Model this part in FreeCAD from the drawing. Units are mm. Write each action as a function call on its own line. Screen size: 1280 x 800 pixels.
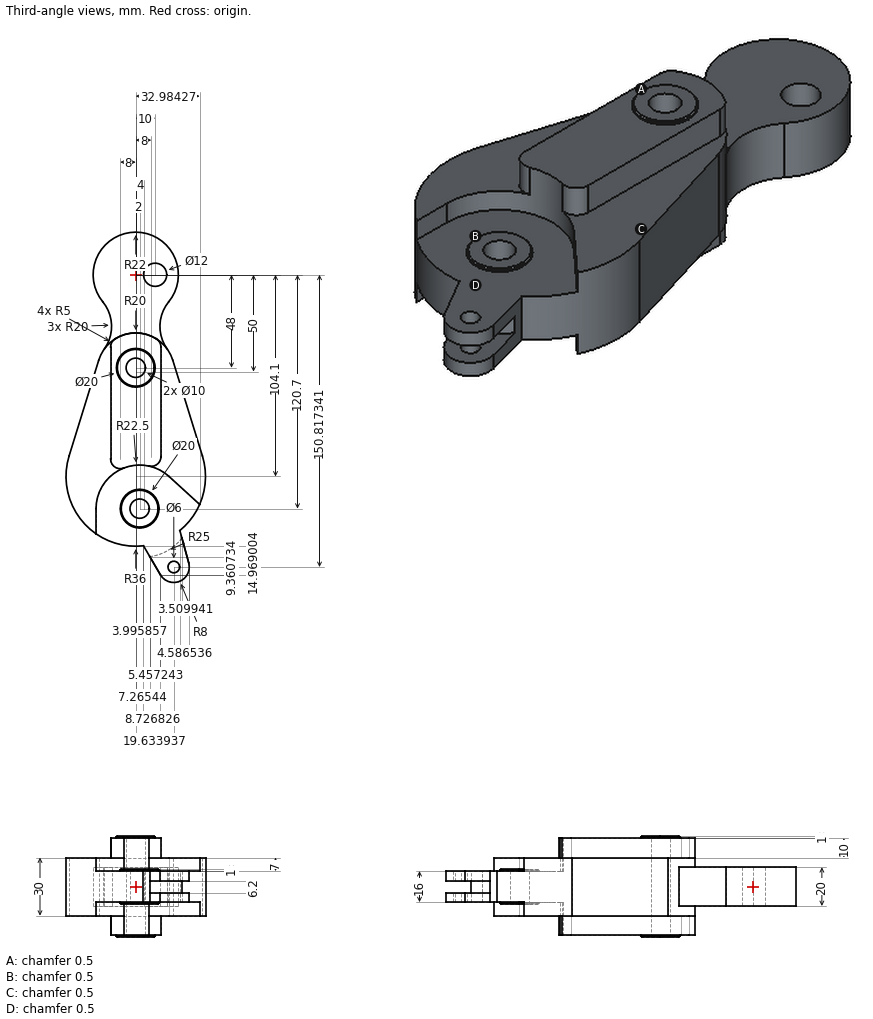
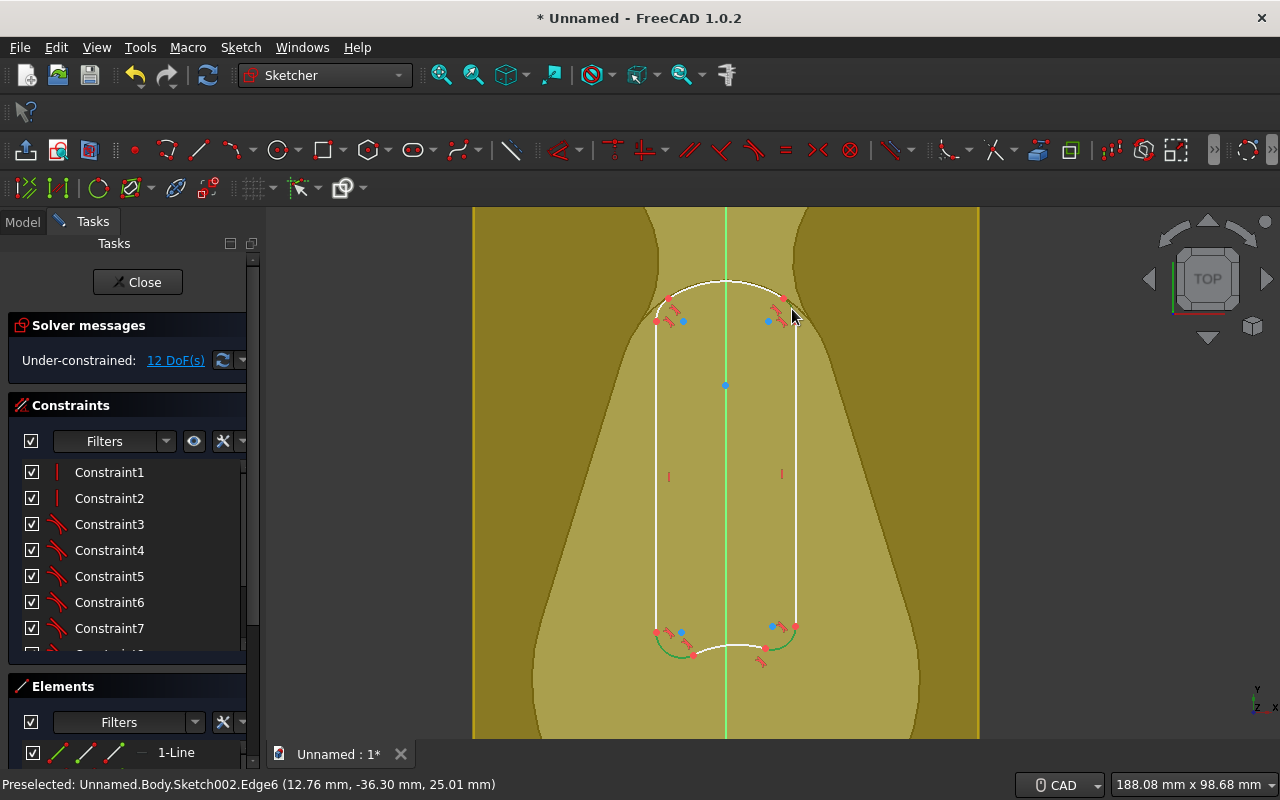
click(659, 309)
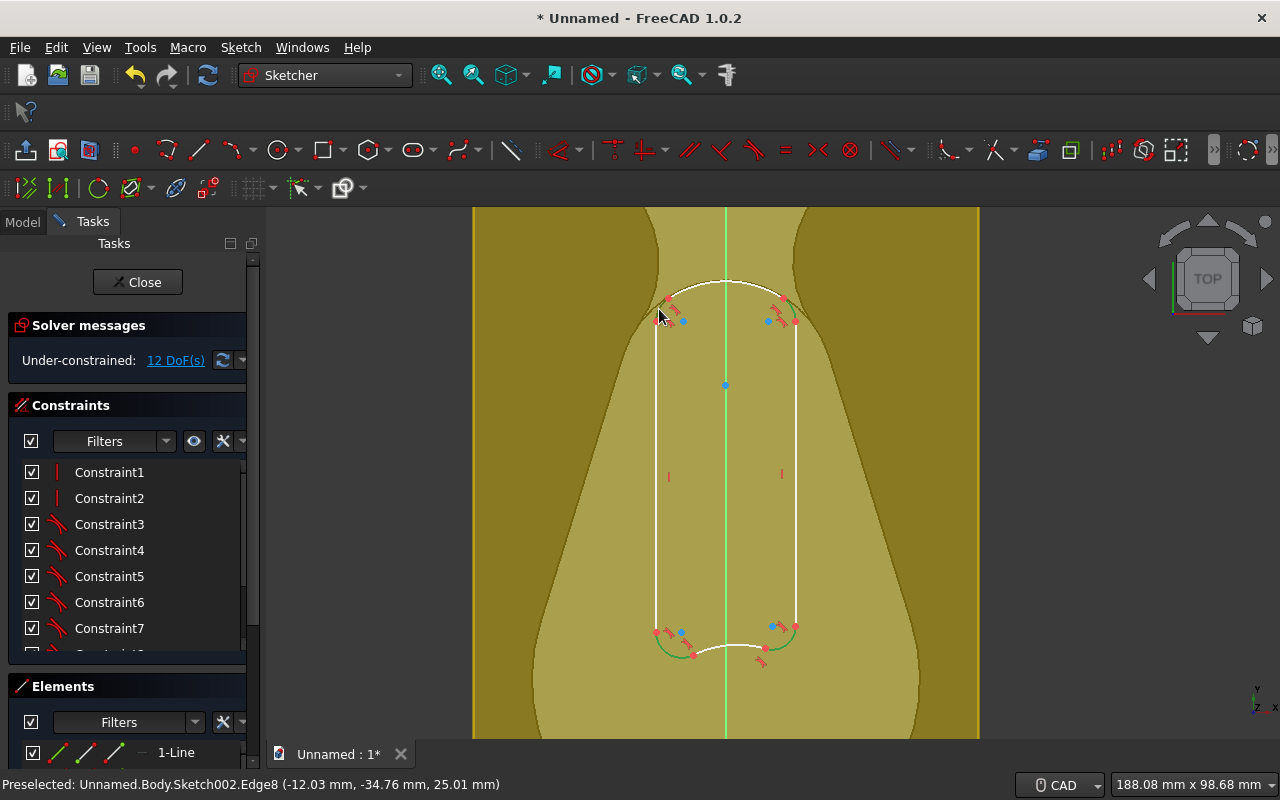
click(786, 150)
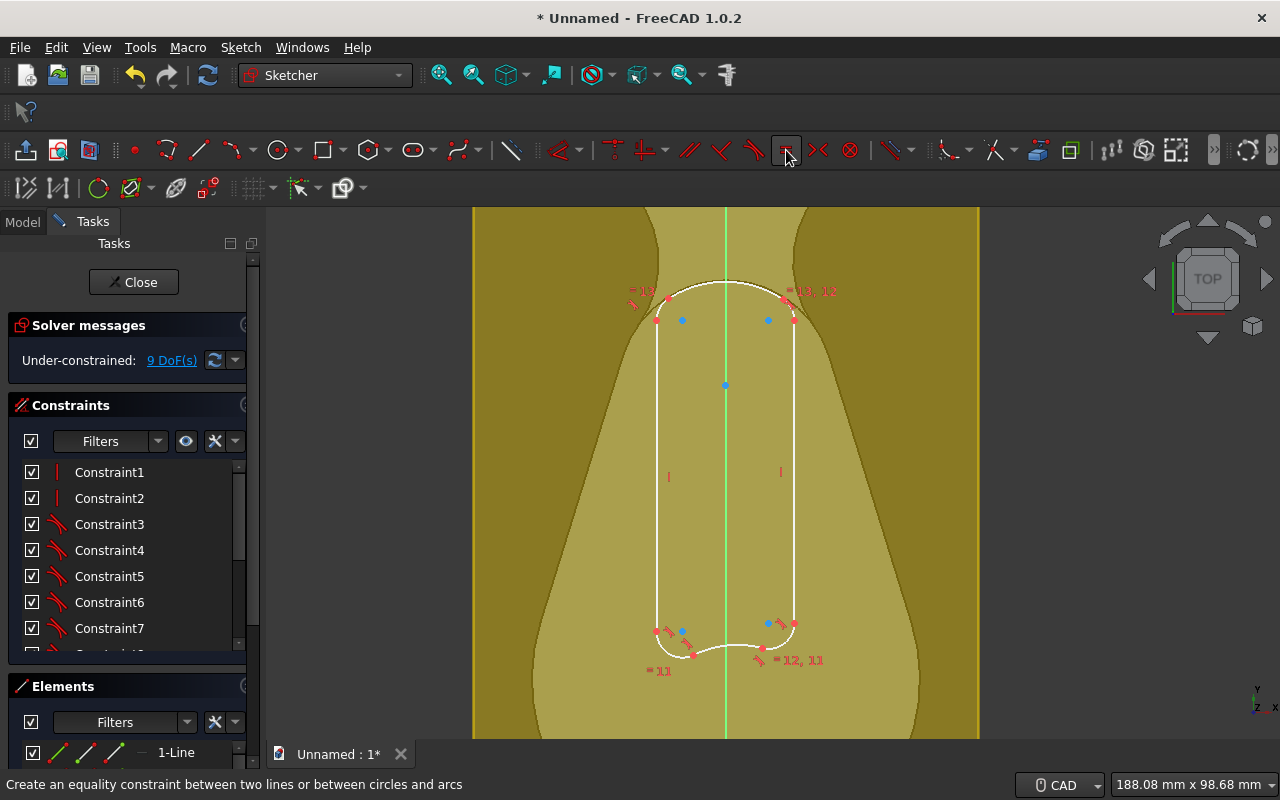
click(725, 385)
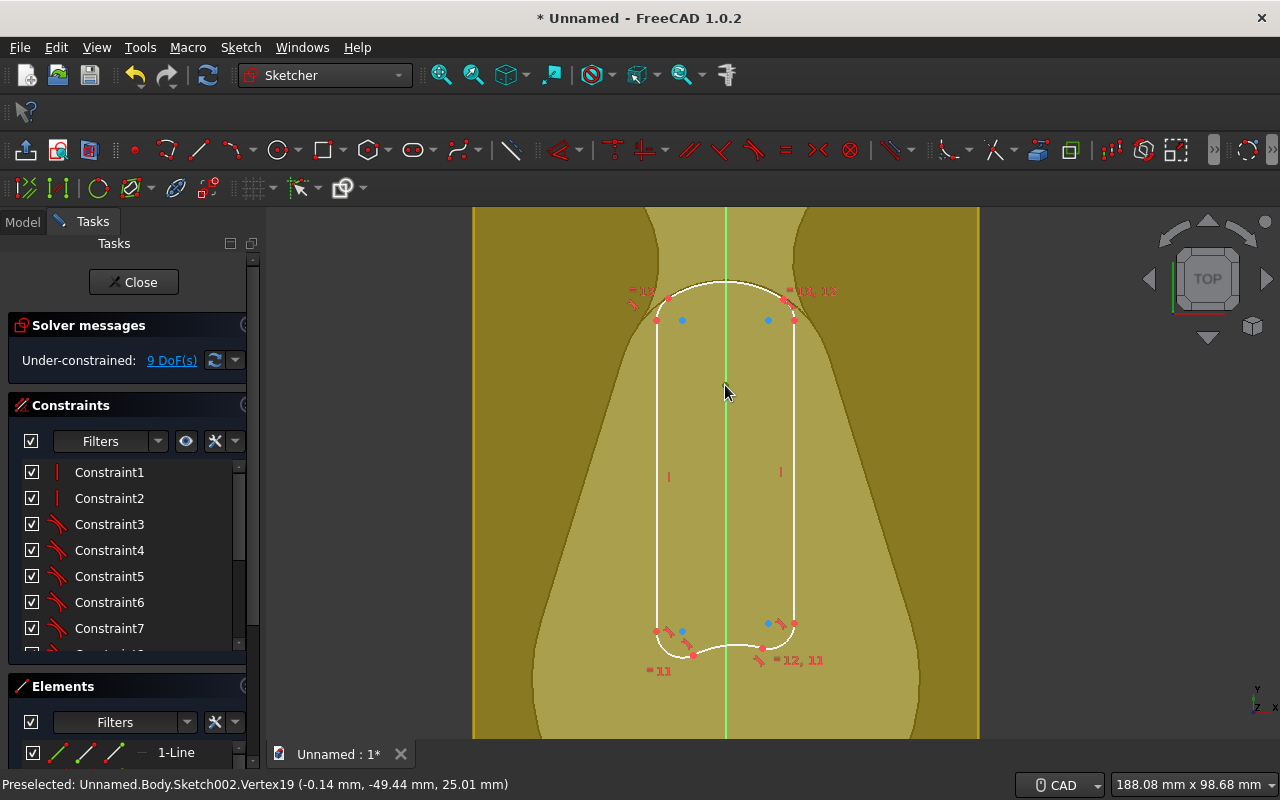
click(726, 677)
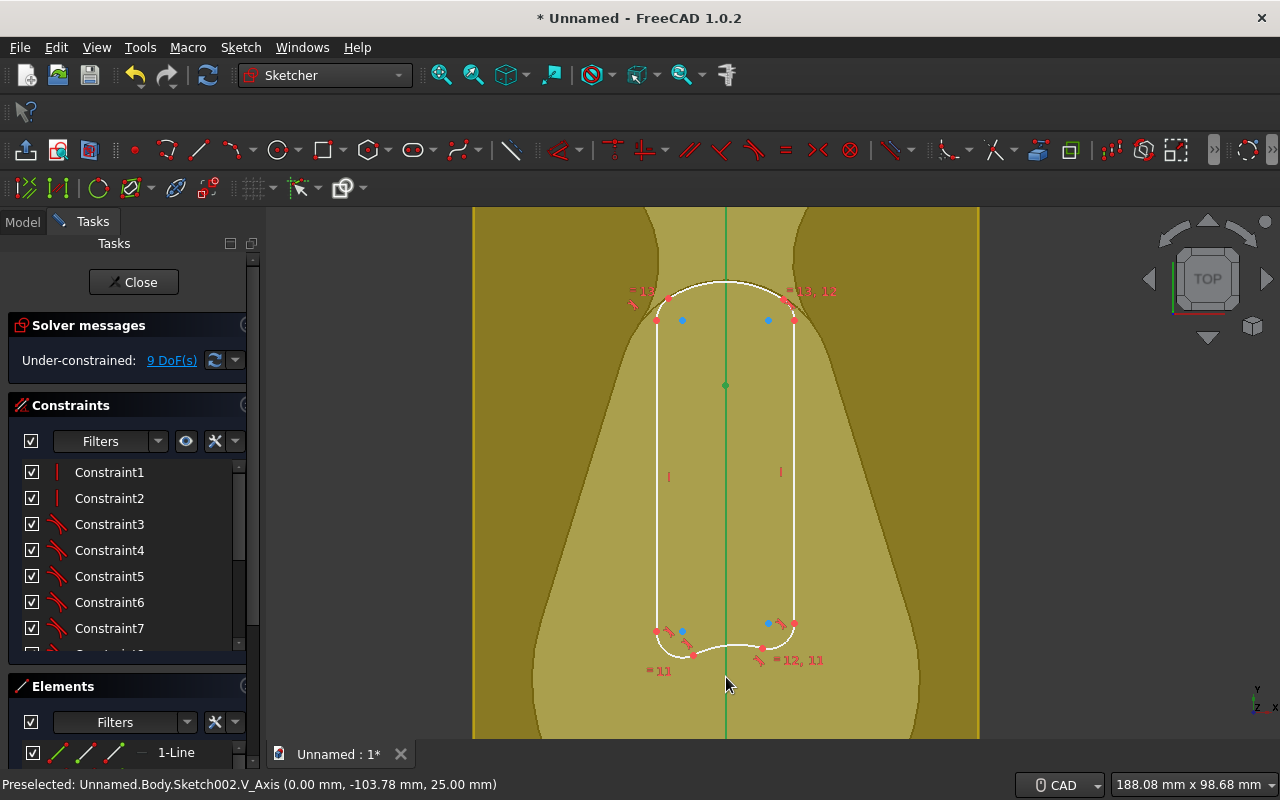
click(614, 150)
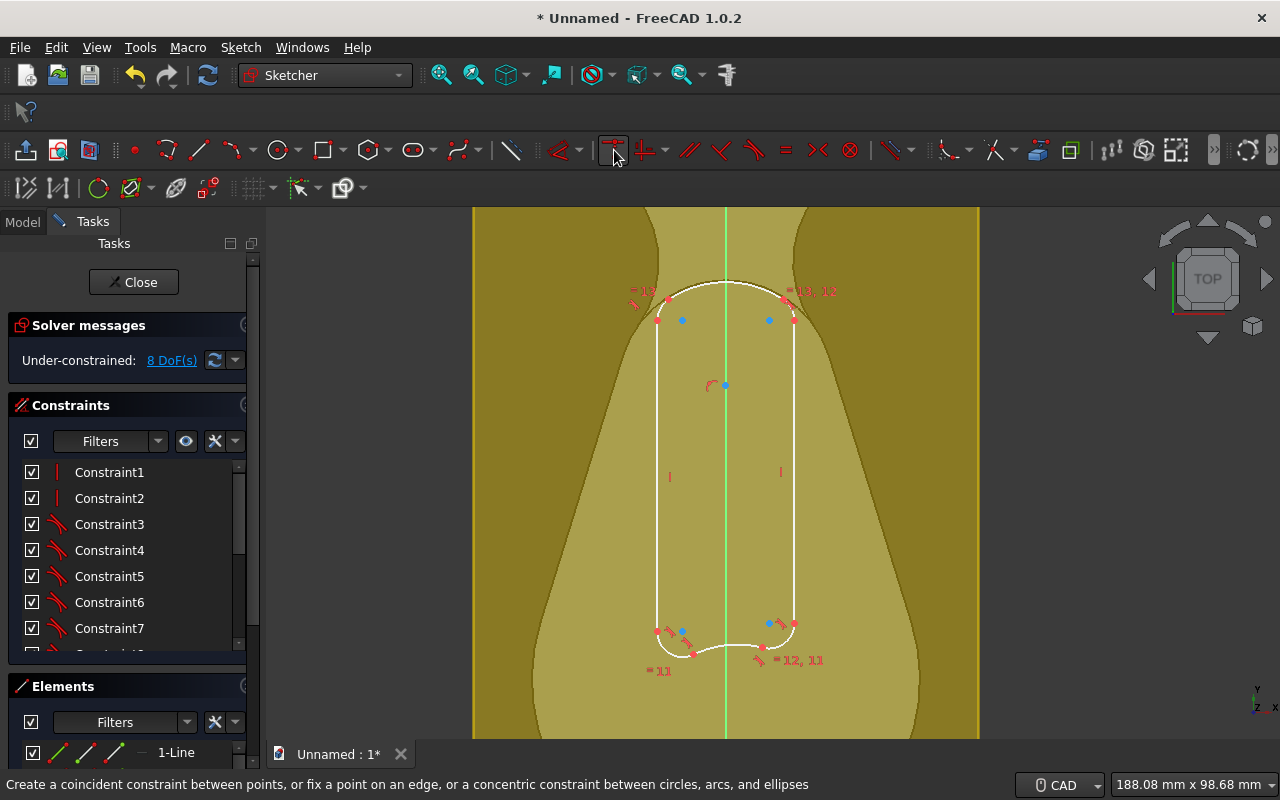
click(558, 150)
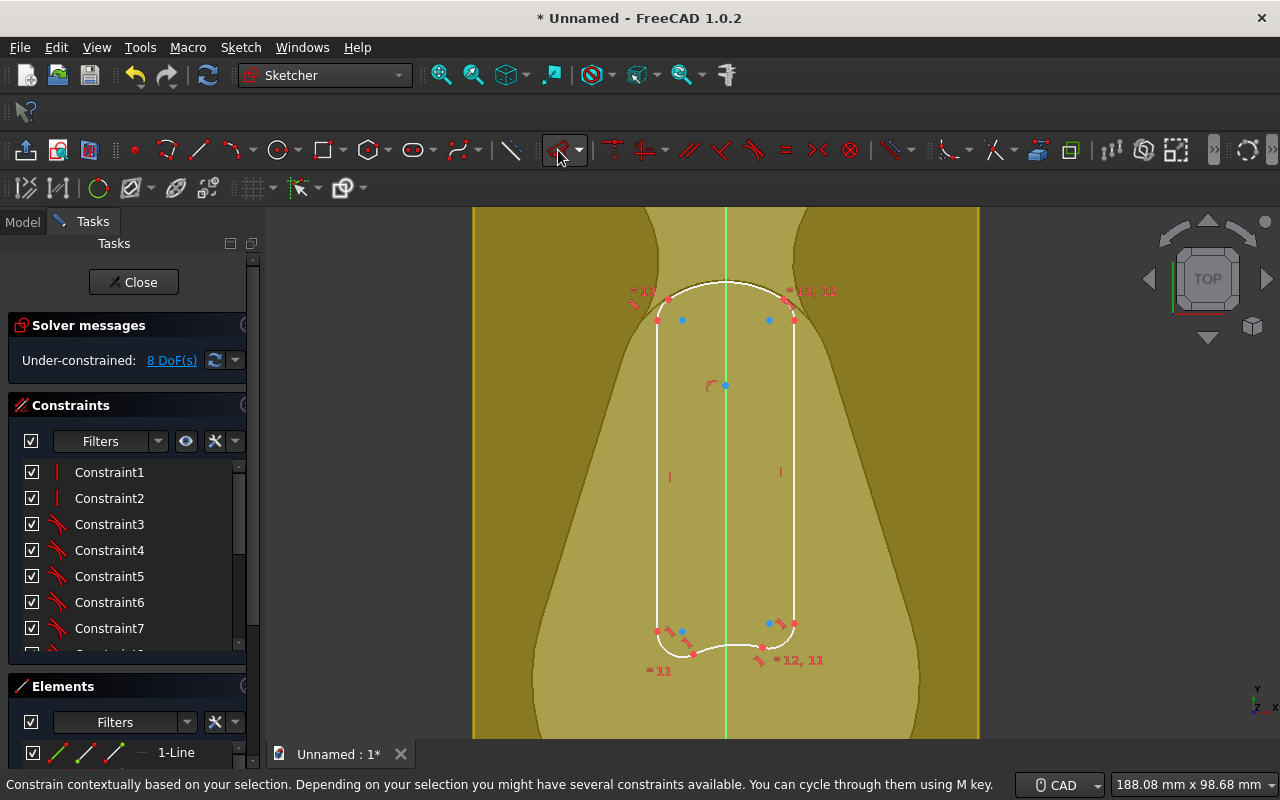
scroll(662, 646, up, 2)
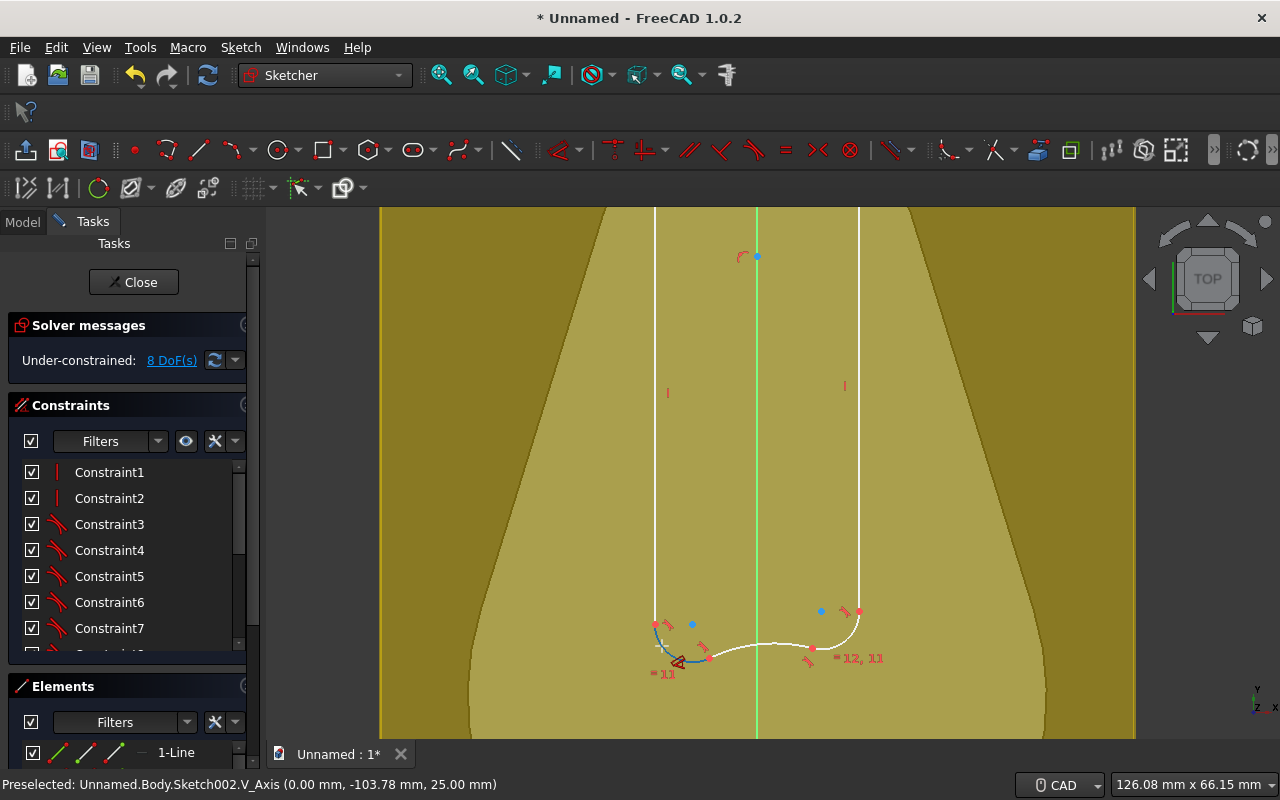
click(662, 646)
click(636, 664)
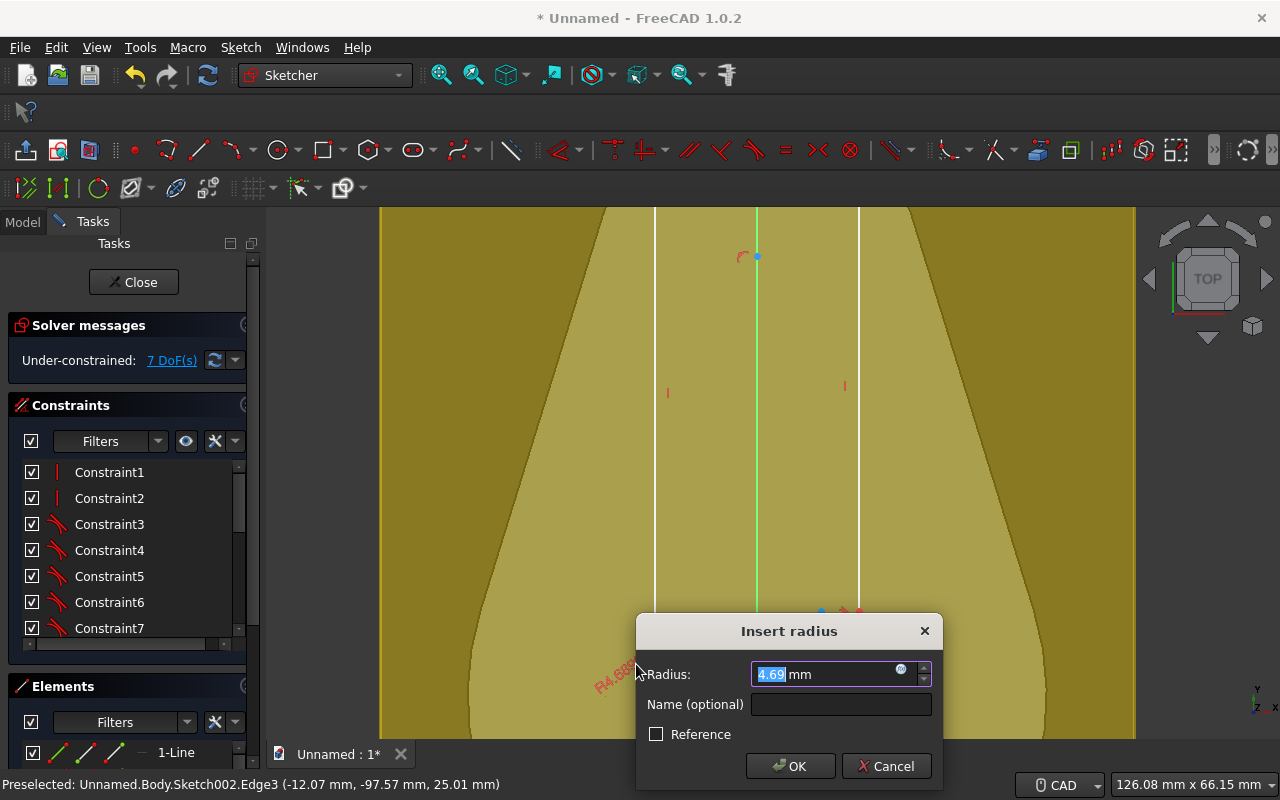
text(5)
key(Return)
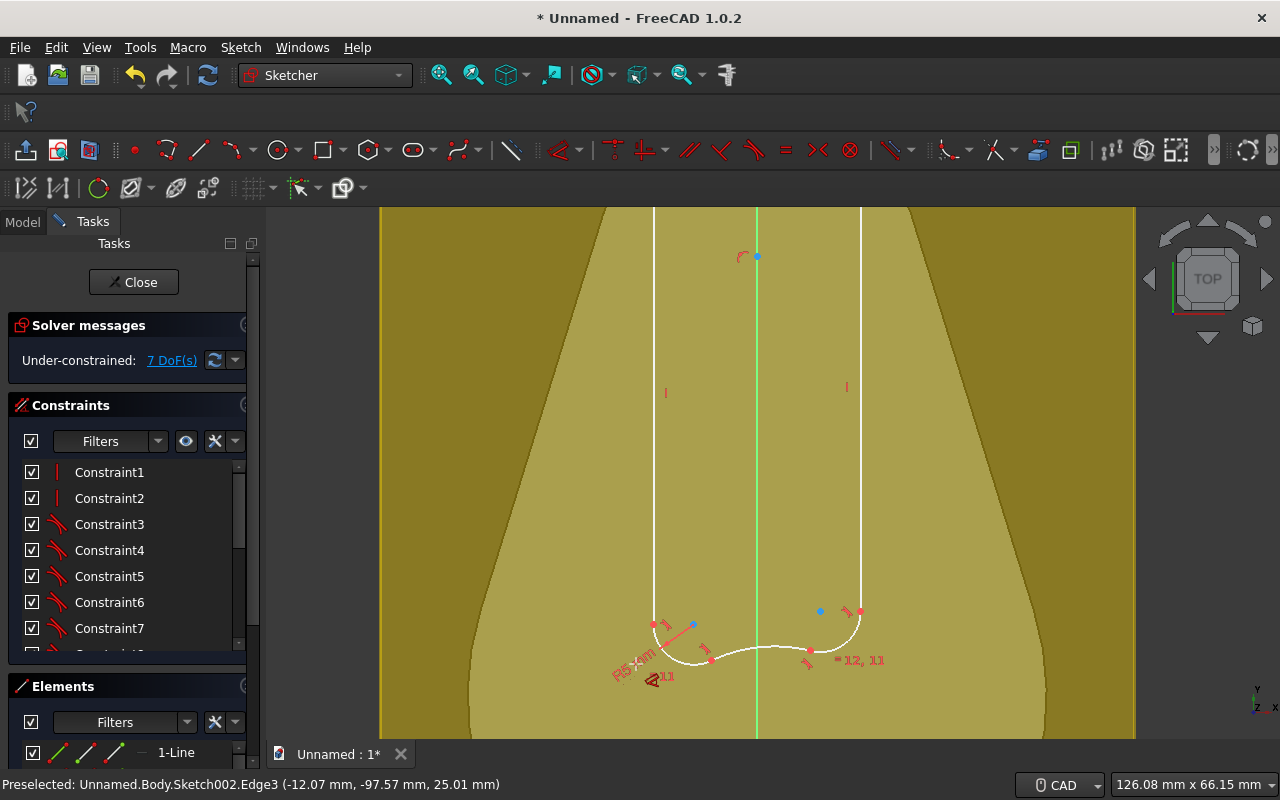
click(780, 647)
click(781, 615)